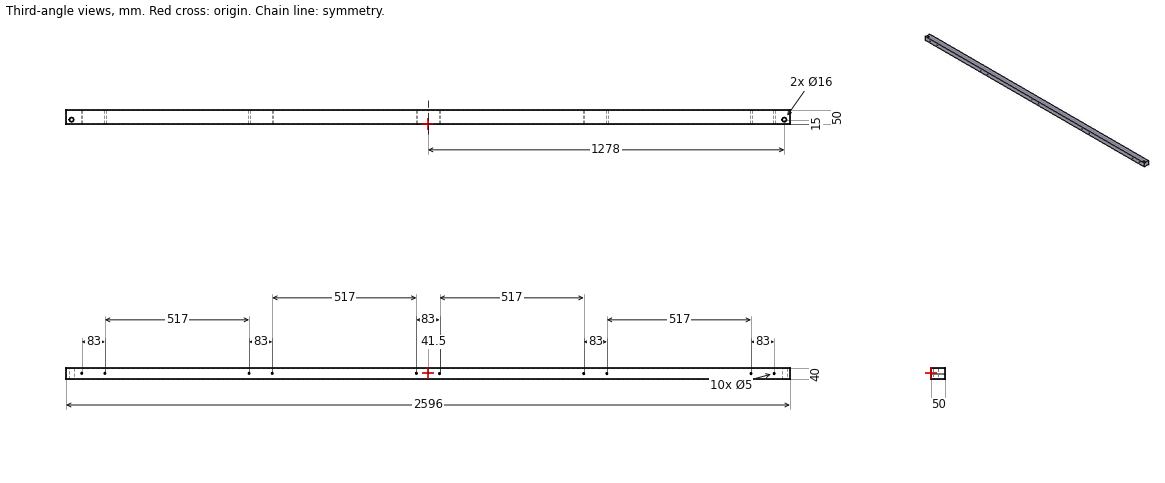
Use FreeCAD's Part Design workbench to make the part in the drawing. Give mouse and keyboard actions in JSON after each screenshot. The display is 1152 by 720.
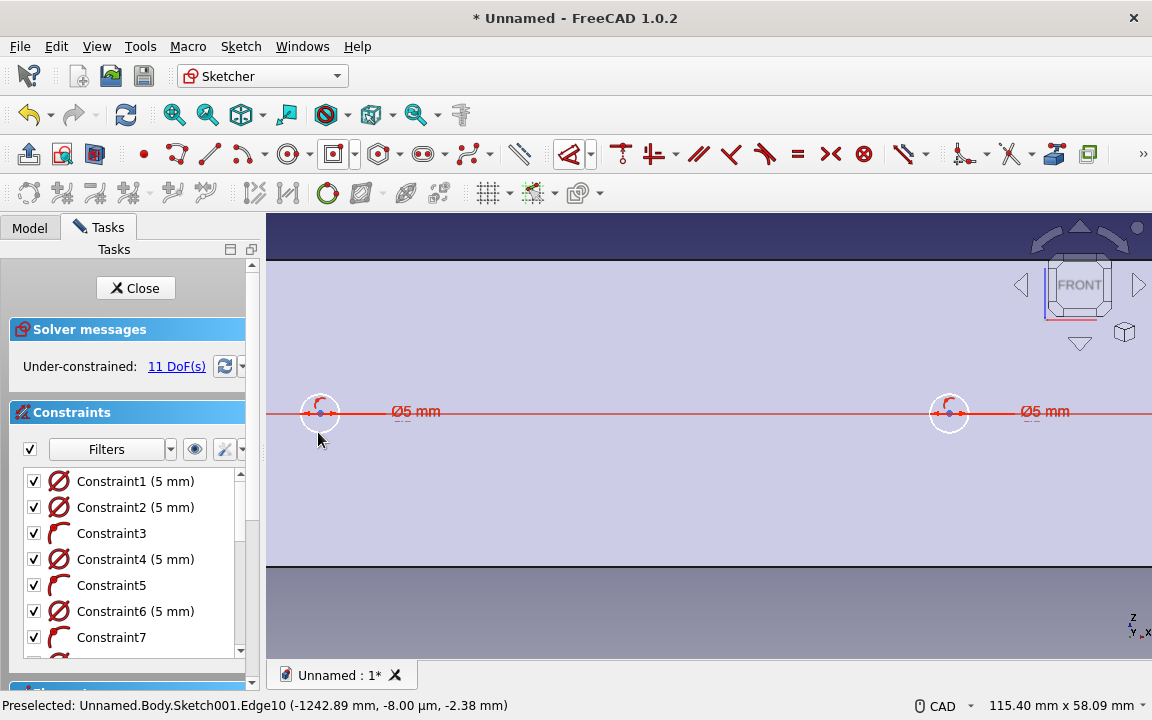
{"action": "scroll", "coordinate": [322, 437], "scroll_direction": "down", "scroll_amount": 17}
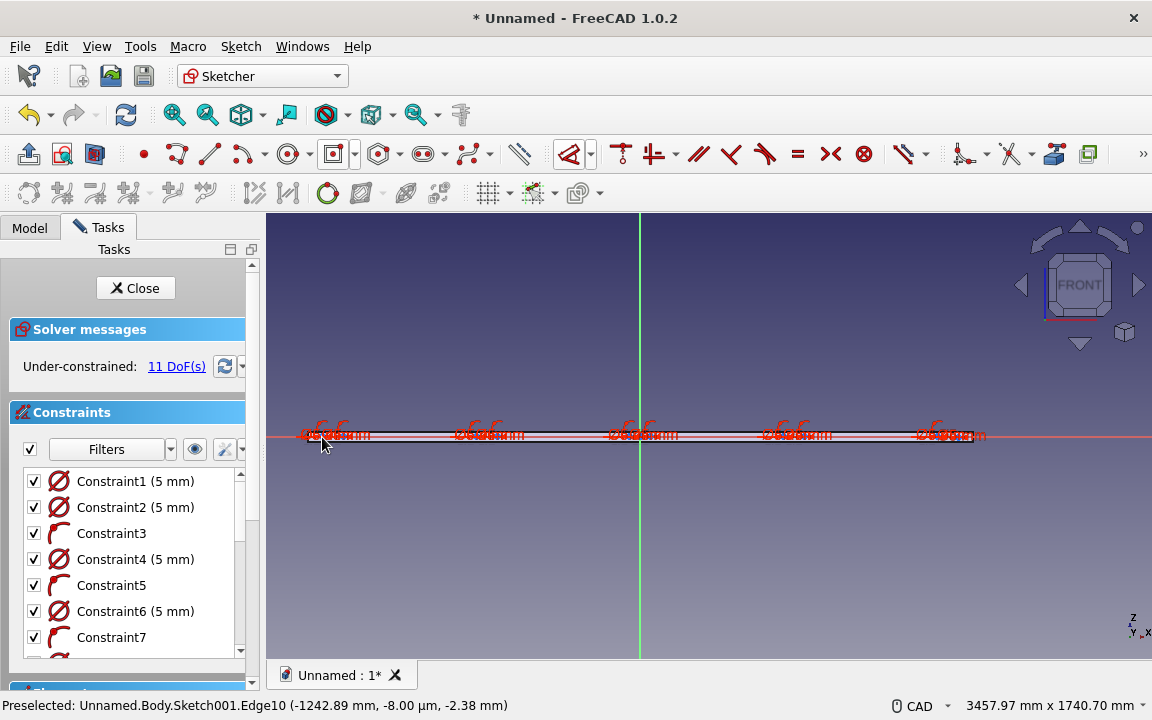
{"action": "left_click", "coordinate": [959, 437]}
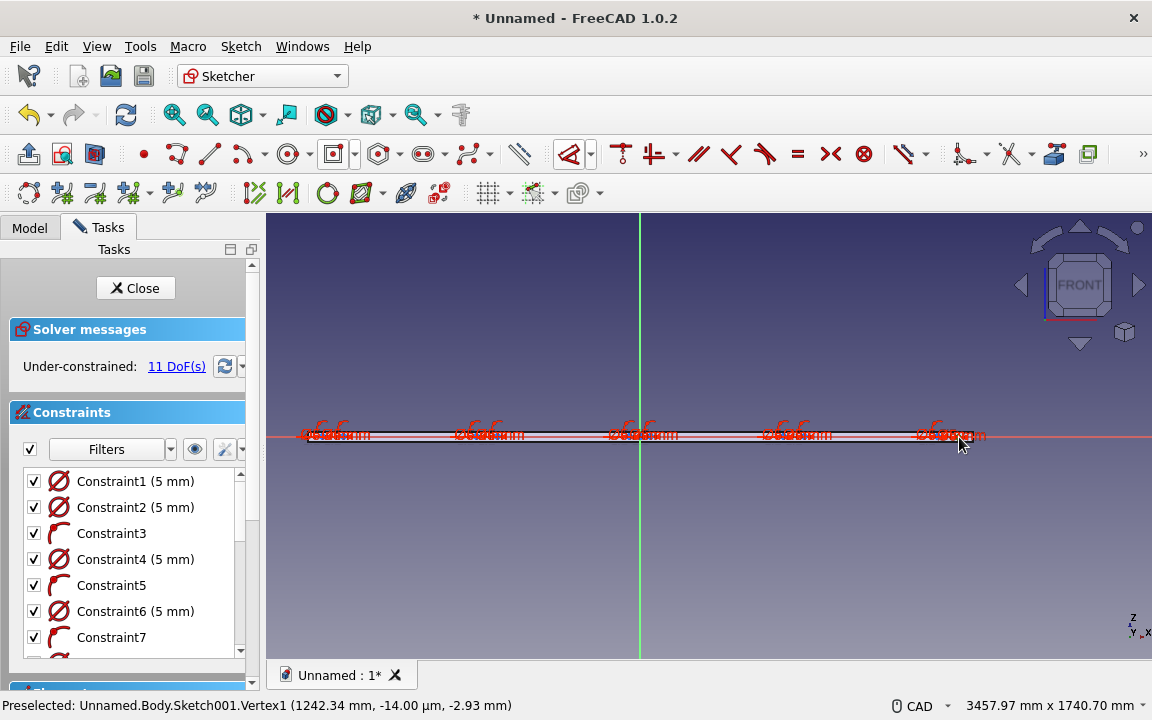
{"action": "left_click", "coordinate": [393, 437]}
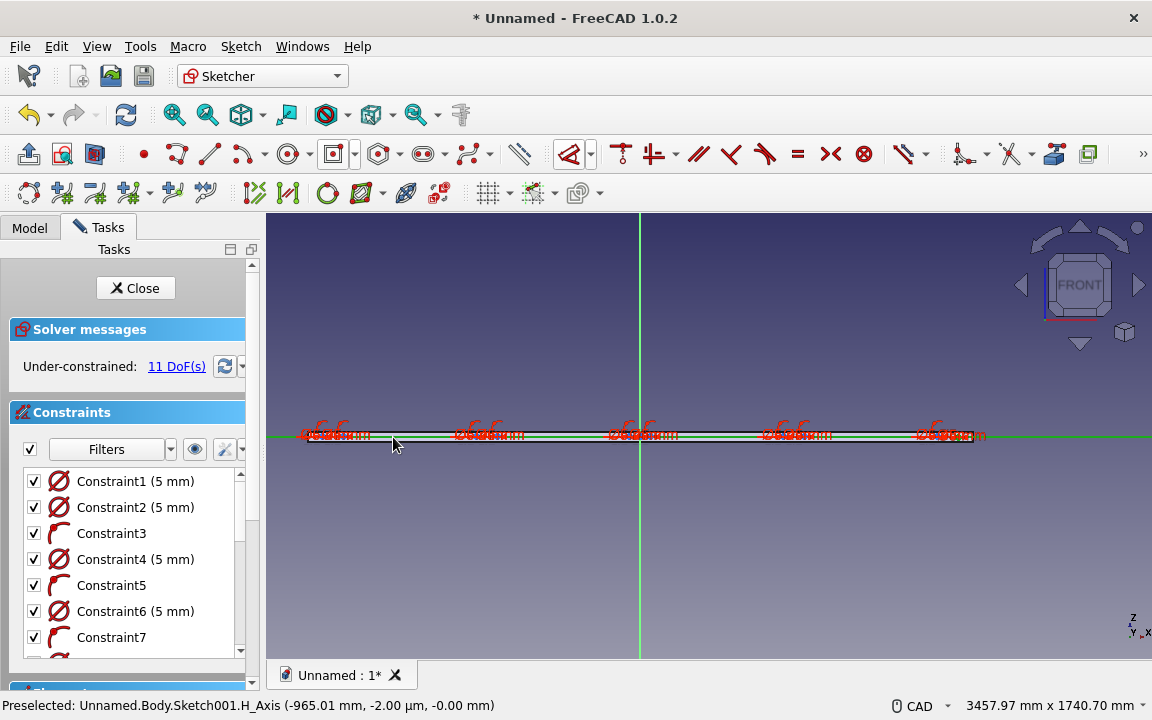
{"action": "left_click", "coordinate": [621, 154]}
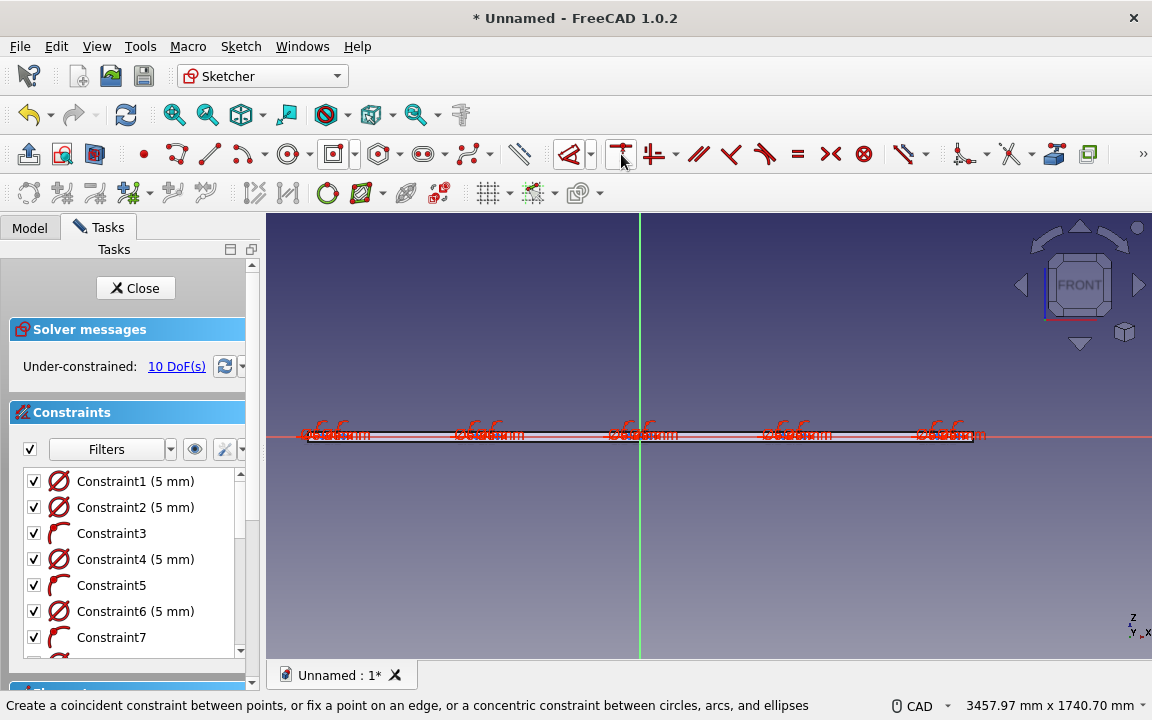
{"action": "scroll", "coordinate": [959, 437], "scroll_direction": "up", "scroll_amount": 4}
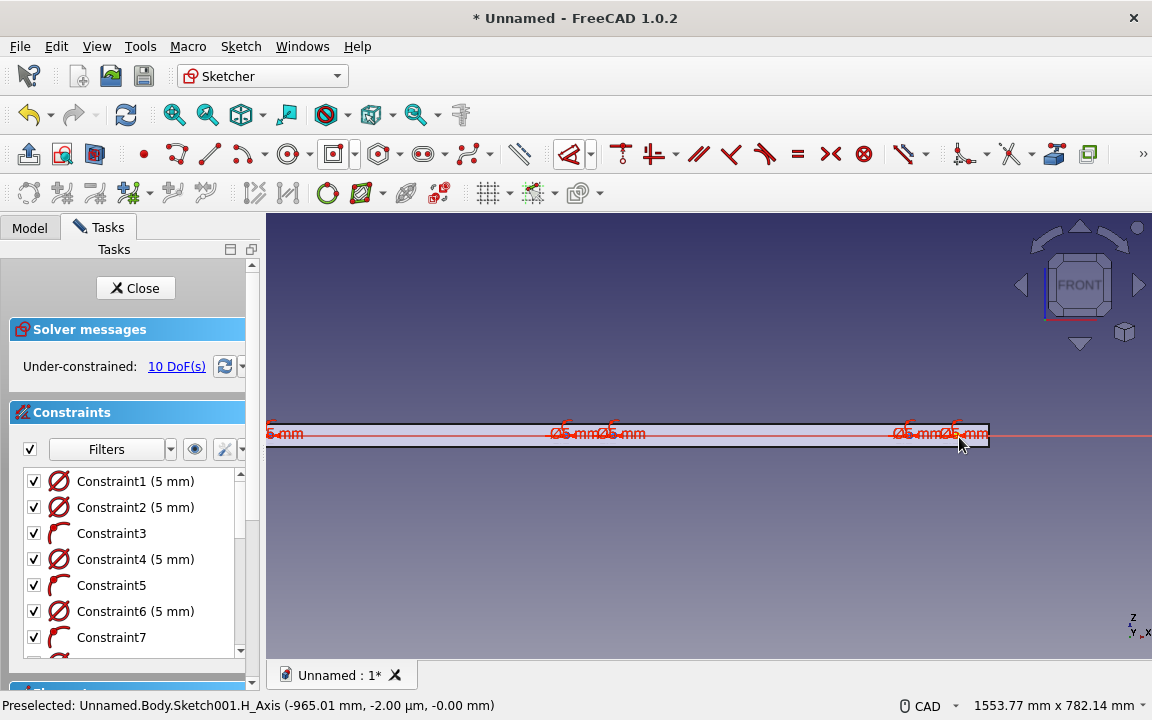
{"action": "left_click", "coordinate": [957, 436]}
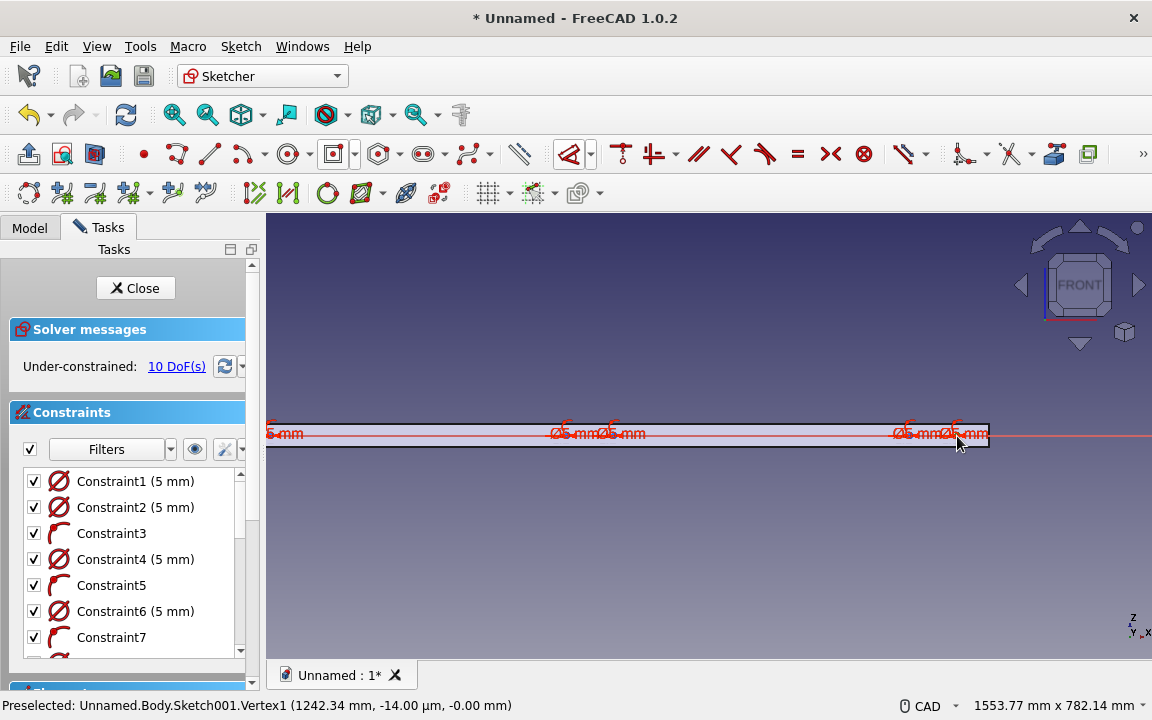
{"action": "left_click", "coordinate": [910, 436]}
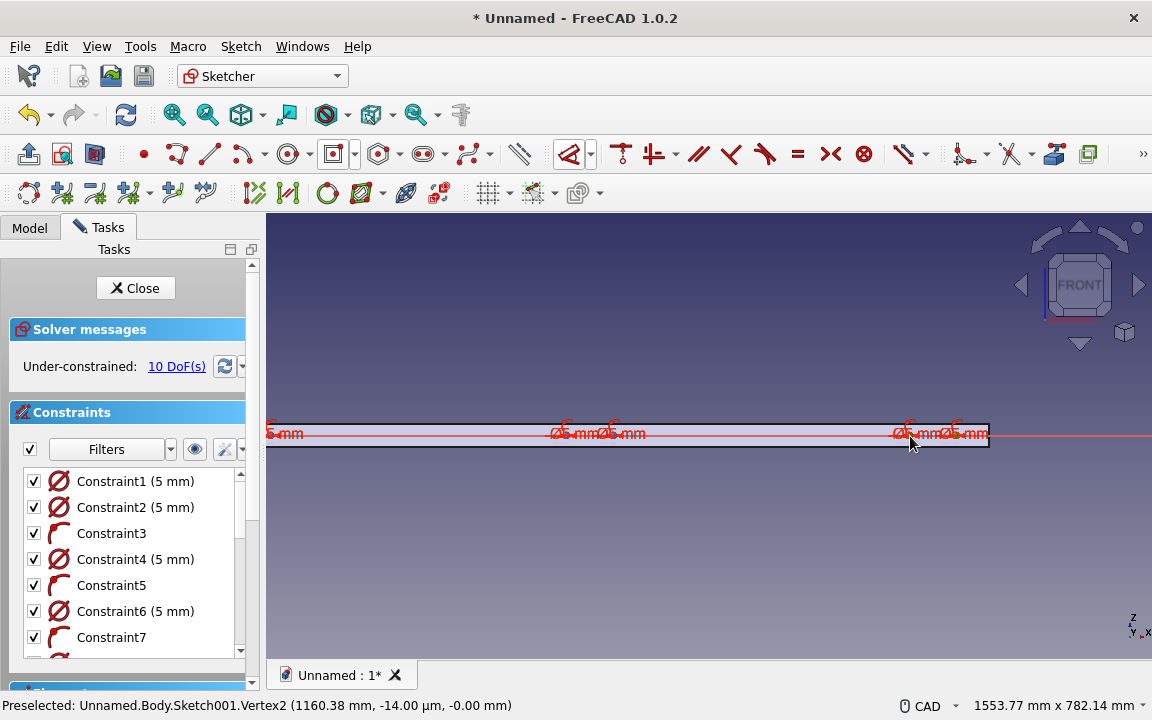
{"action": "left_click", "coordinate": [590, 154]}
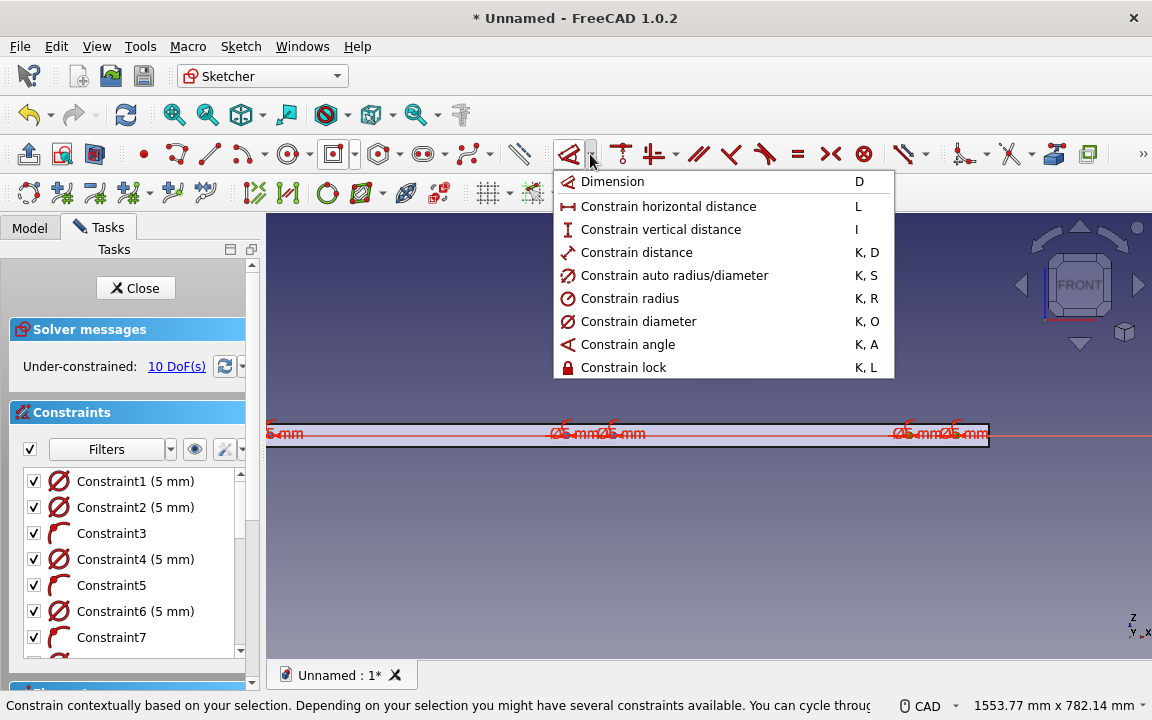
{"action": "left_click", "coordinate": [724, 206]}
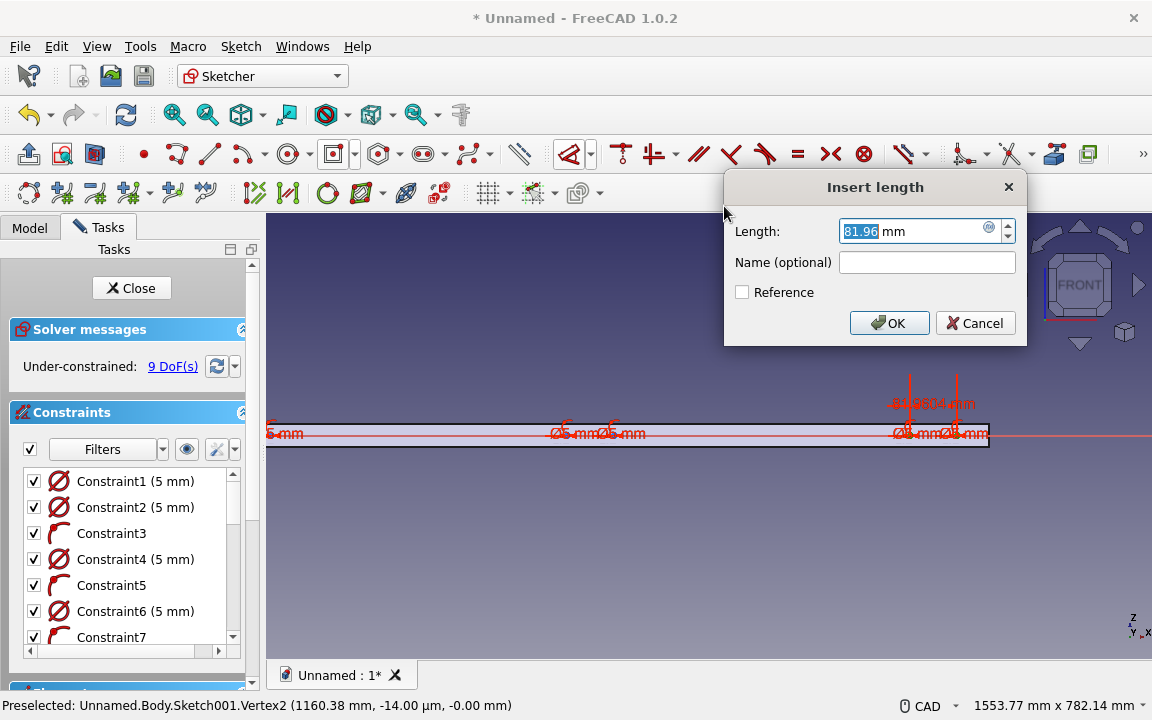
{"action": "type", "text": "83"}
{"action": "key", "text": "Return"}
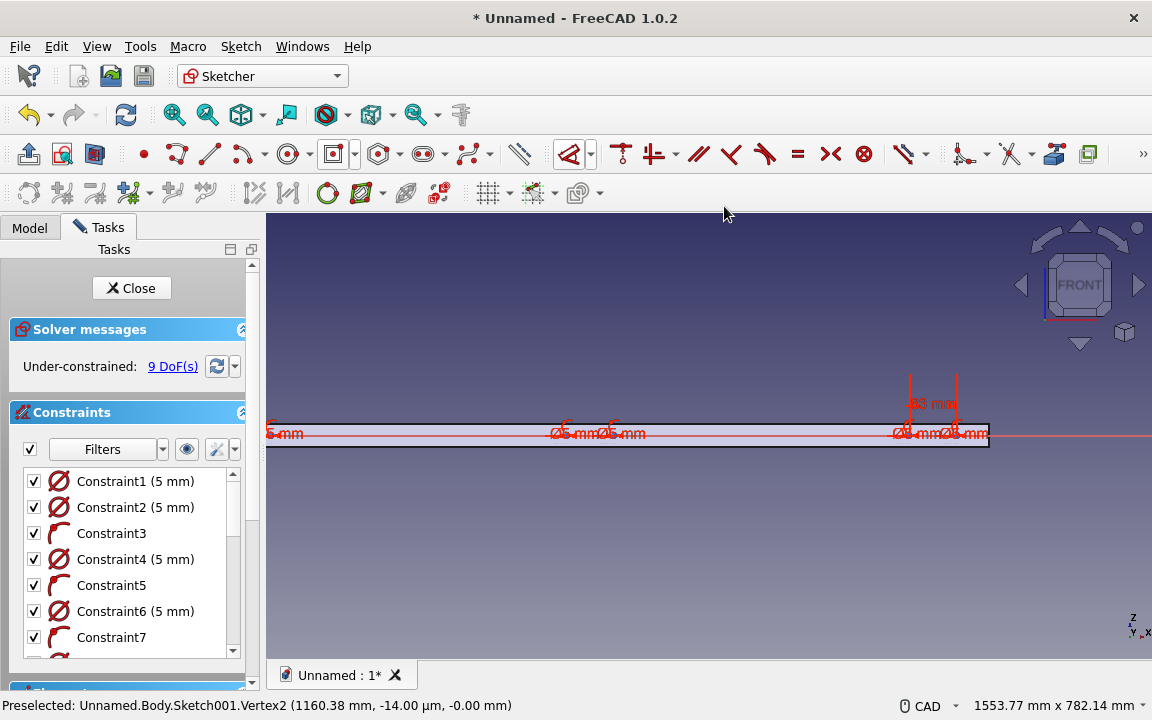
{"action": "left_click", "coordinate": [614, 436]}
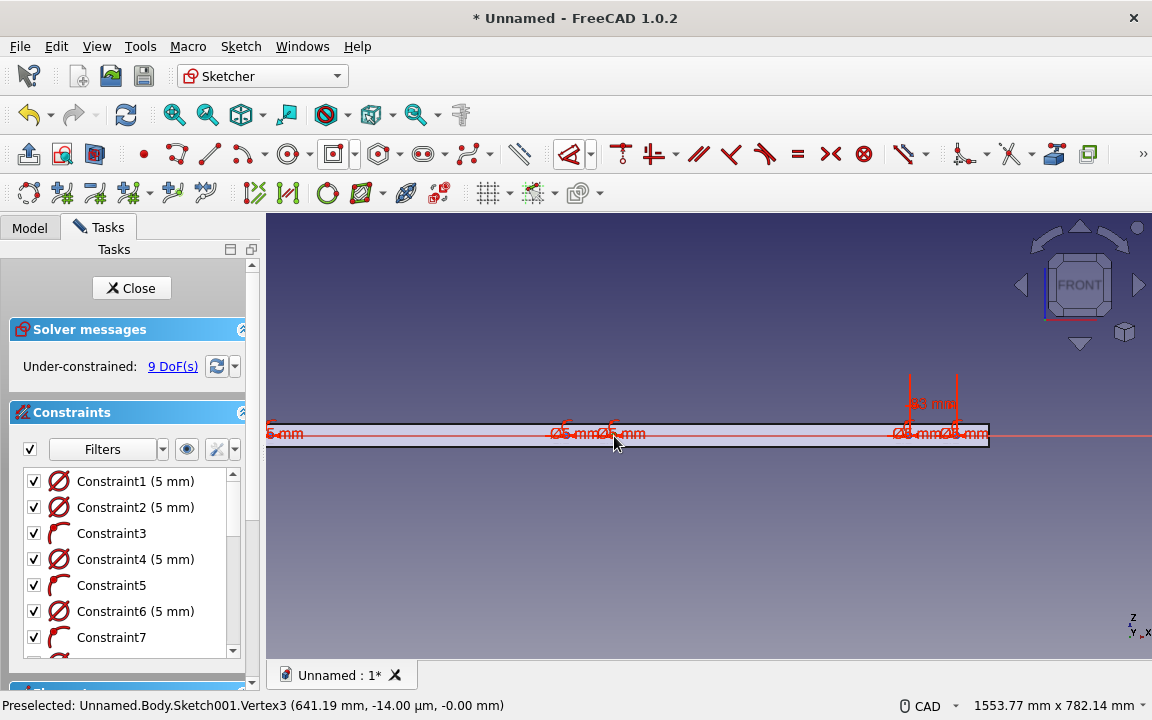
{"action": "left_click", "coordinate": [568, 436]}